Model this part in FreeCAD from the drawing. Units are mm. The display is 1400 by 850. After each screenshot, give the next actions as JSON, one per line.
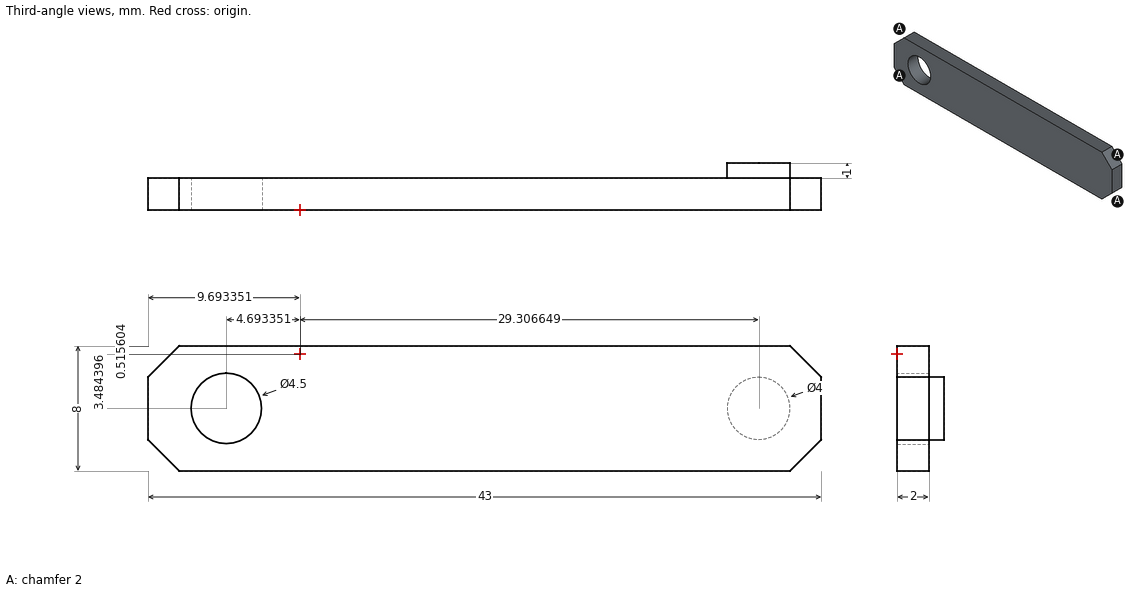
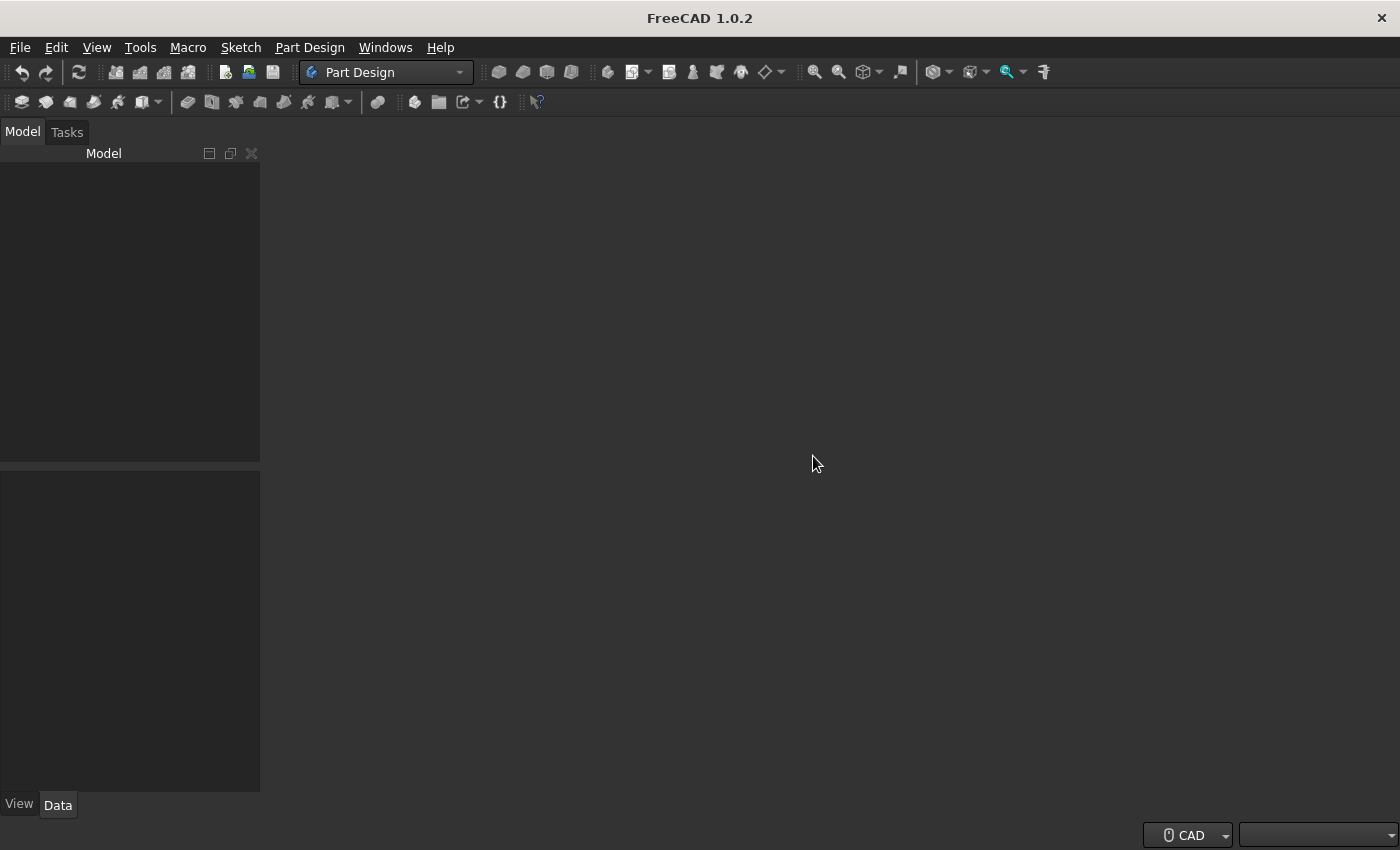
{"action": "left_click", "coordinate": [226, 72]}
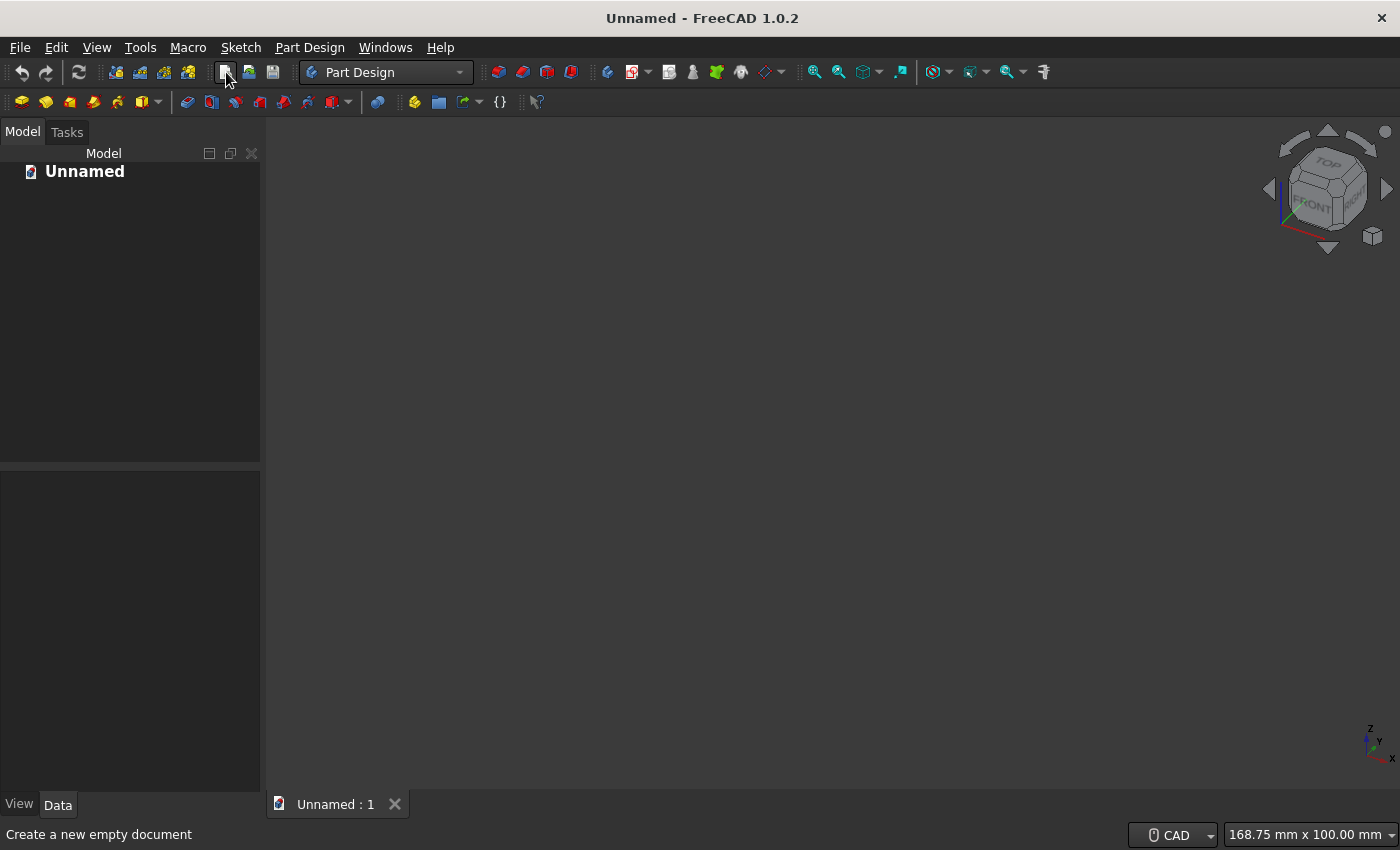
{"action": "left_click", "coordinate": [632, 72]}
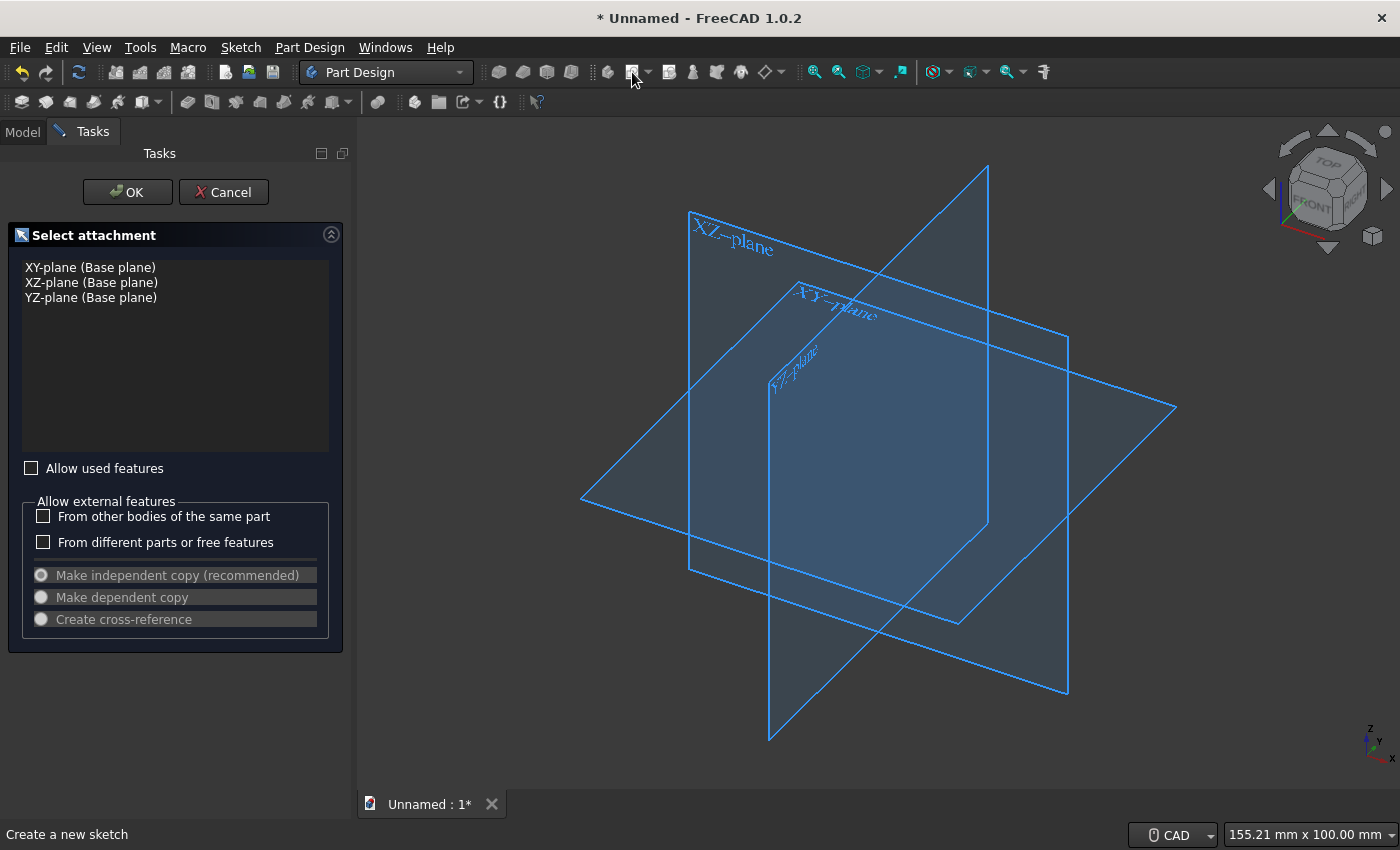
{"action": "left_click", "coordinate": [82, 282]}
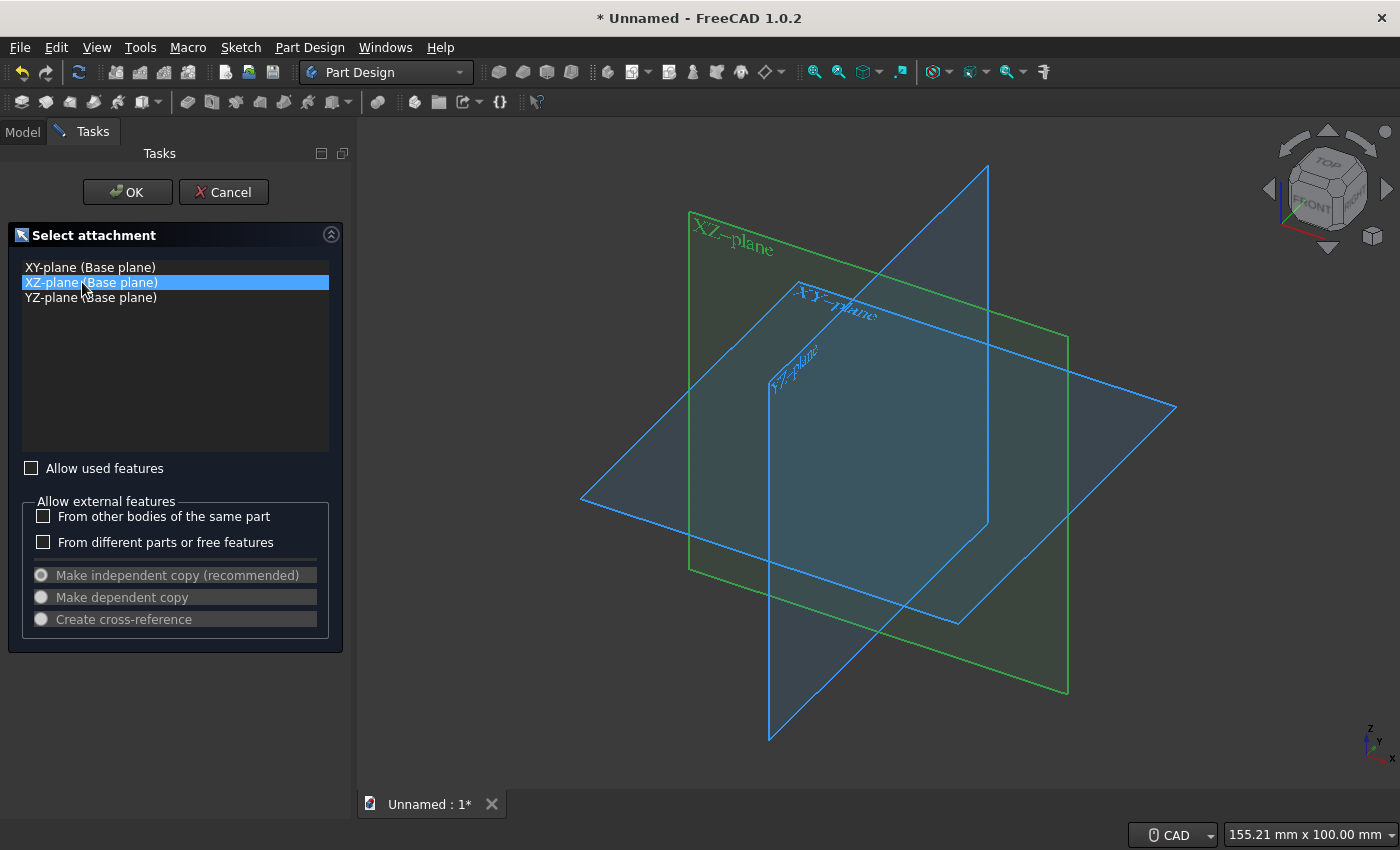
{"action": "left_click", "coordinate": [128, 192]}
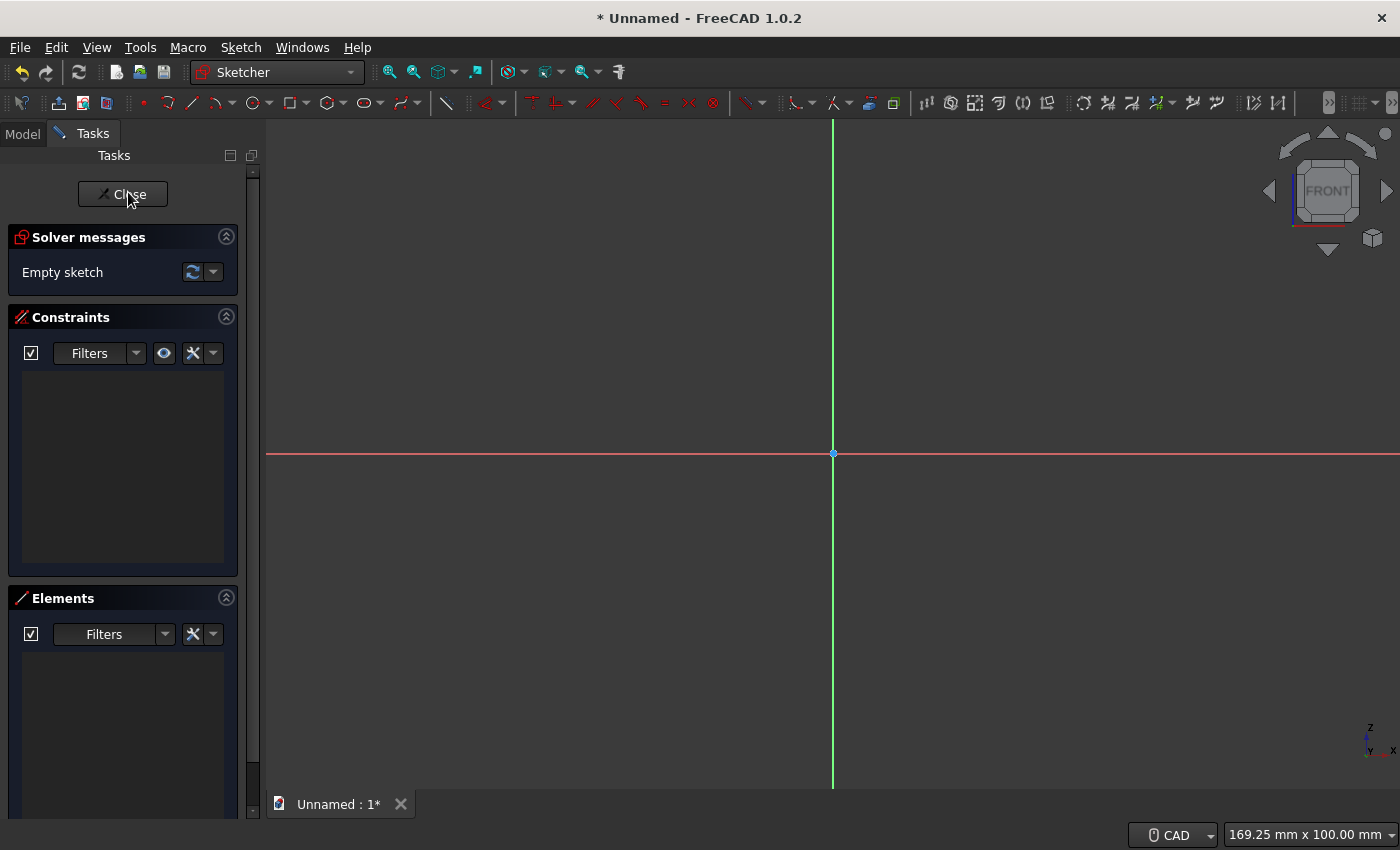
{"action": "scroll", "coordinate": [1033, 496], "scroll_direction": "up", "scroll_amount": 4}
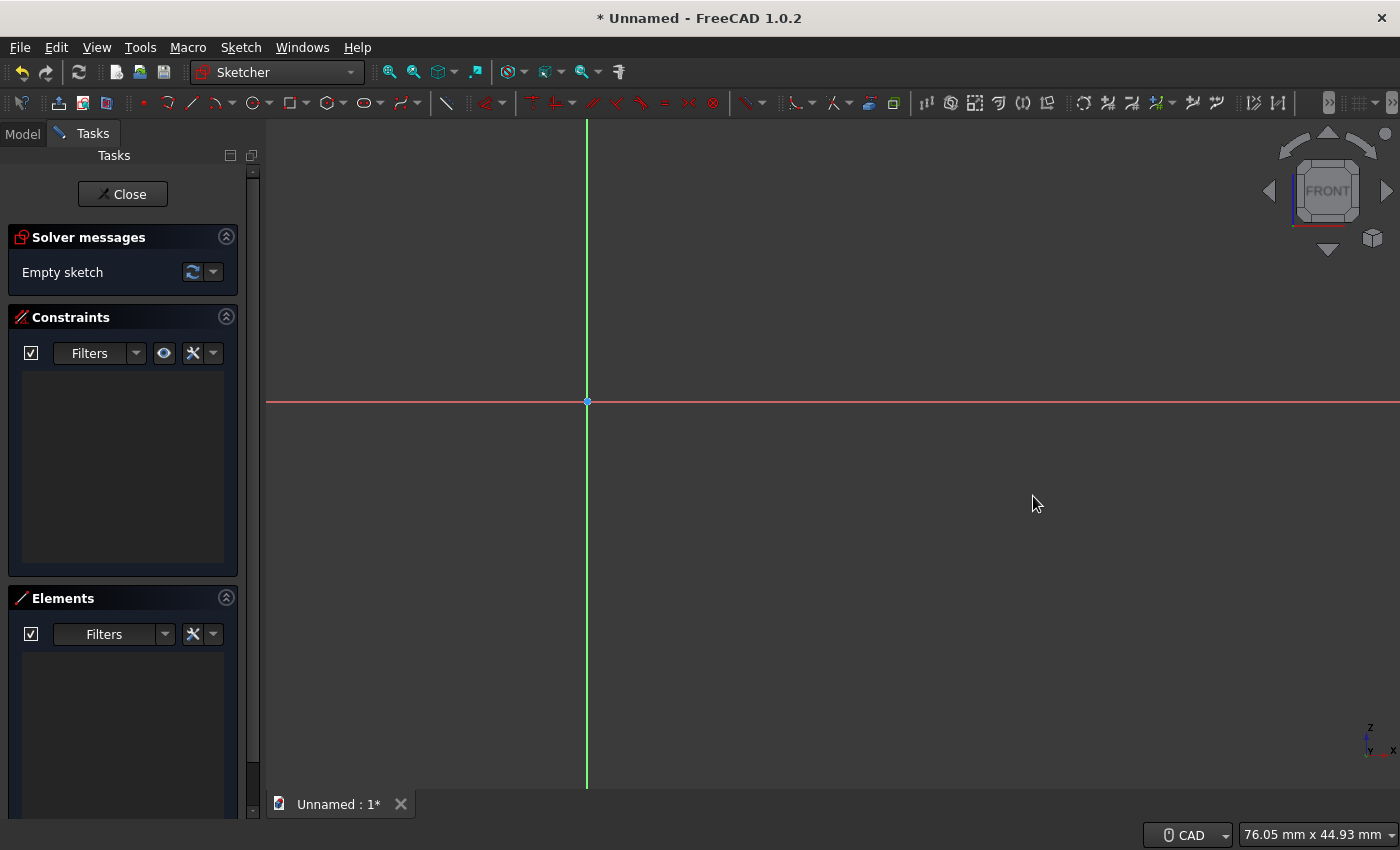
{"action": "left_click", "coordinate": [290, 104]}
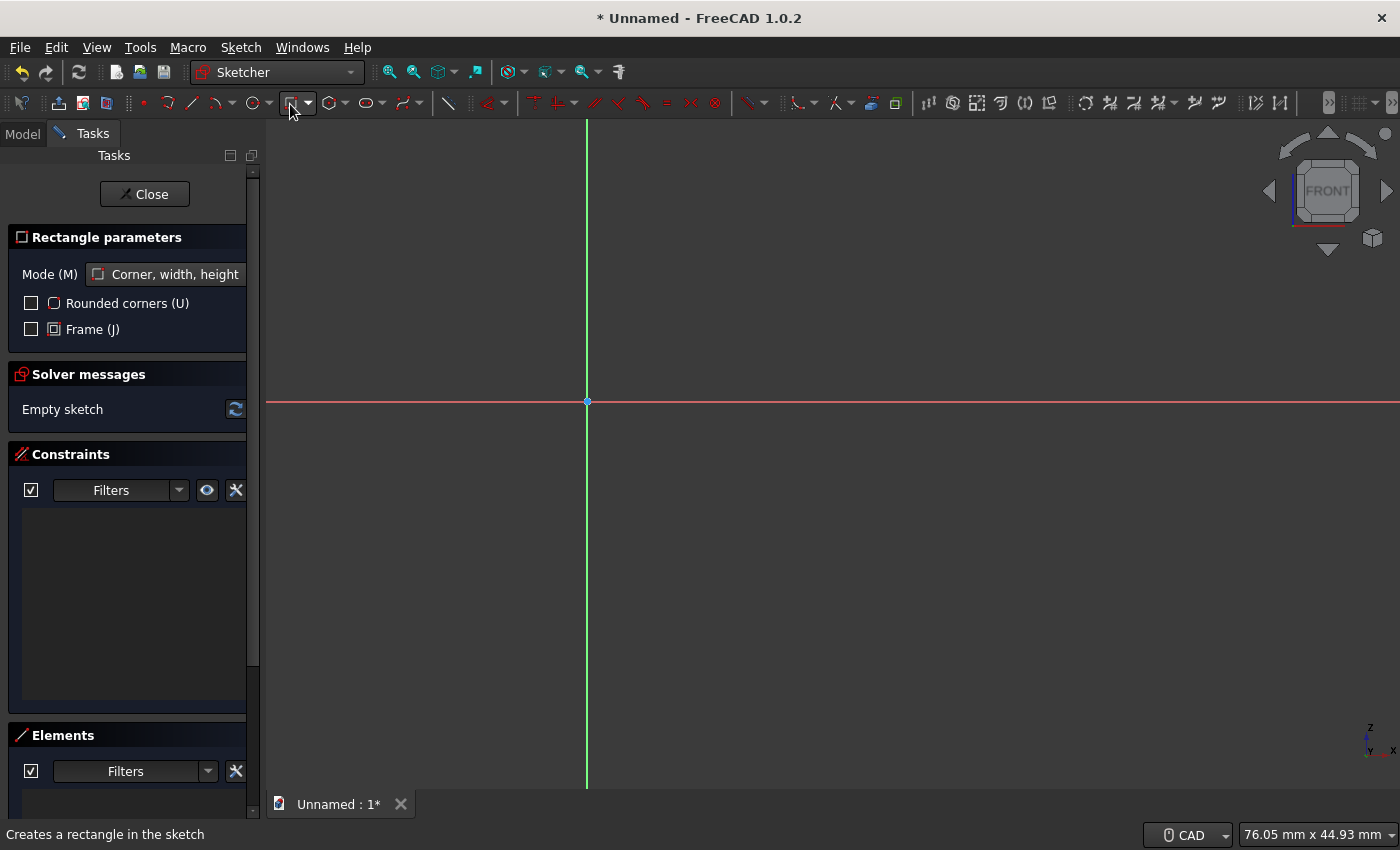
{"action": "scroll", "coordinate": [443, 394], "scroll_direction": "up", "scroll_amount": 4}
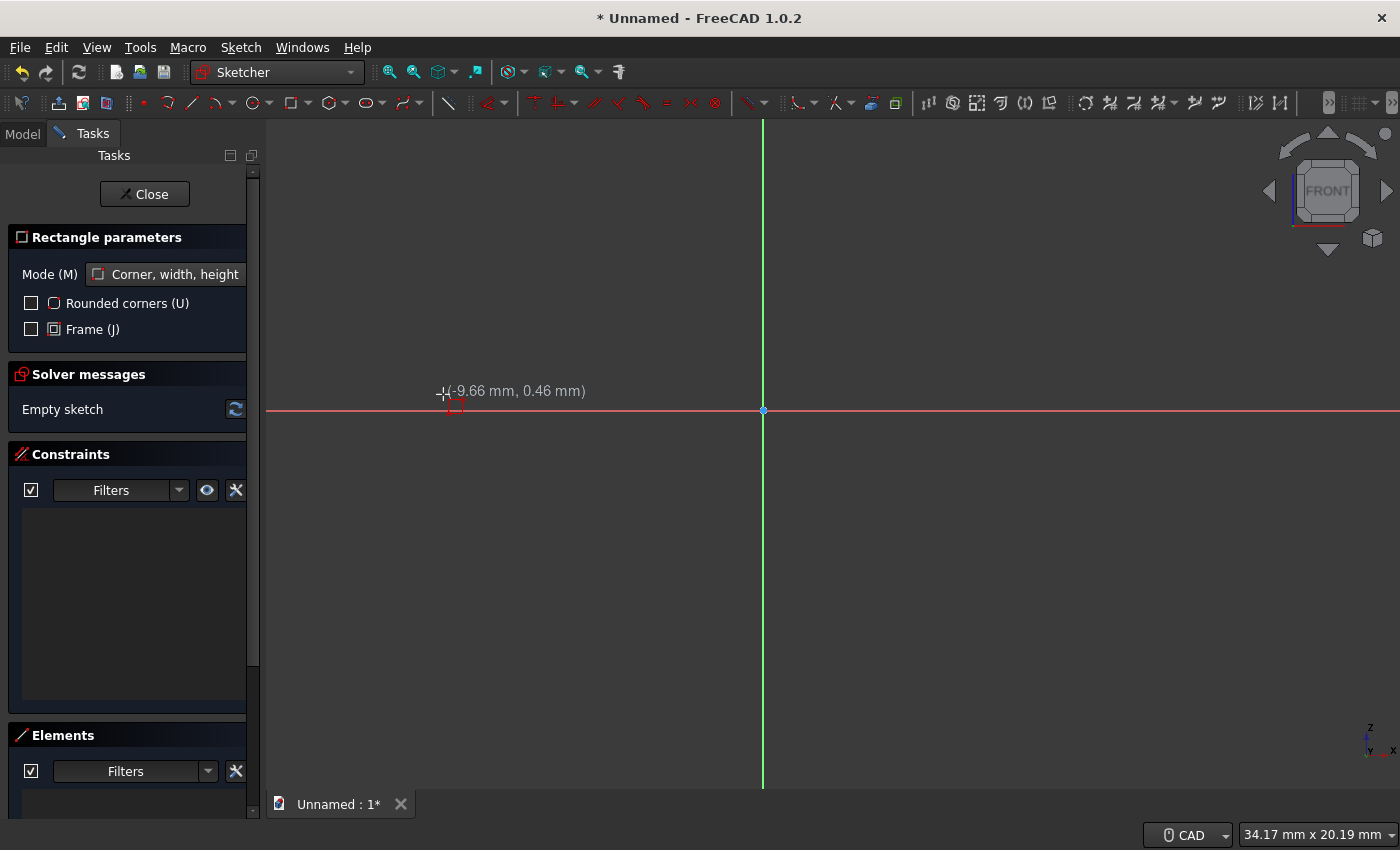
{"action": "left_click", "coordinate": [442, 394]}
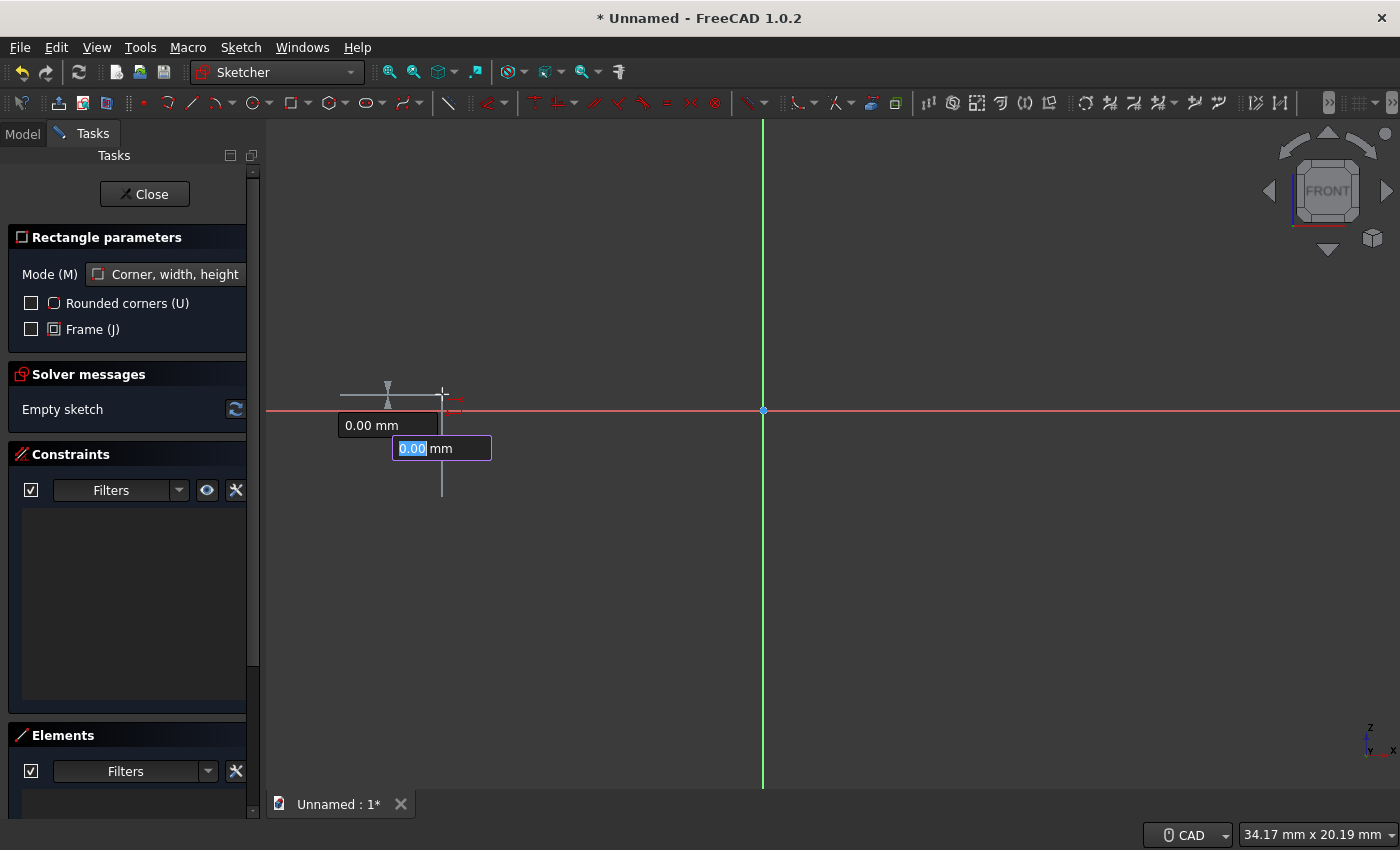
{"action": "scroll", "coordinate": [446, 395], "scroll_direction": "down", "scroll_amount": 4}